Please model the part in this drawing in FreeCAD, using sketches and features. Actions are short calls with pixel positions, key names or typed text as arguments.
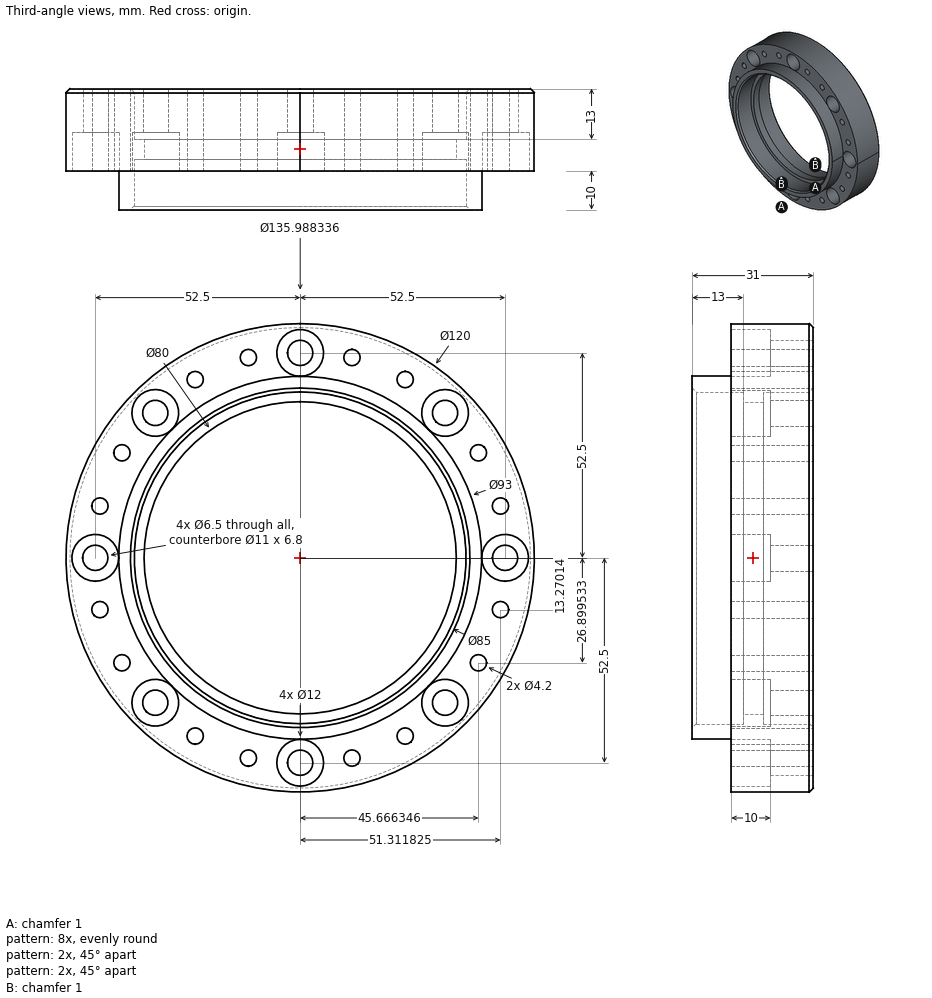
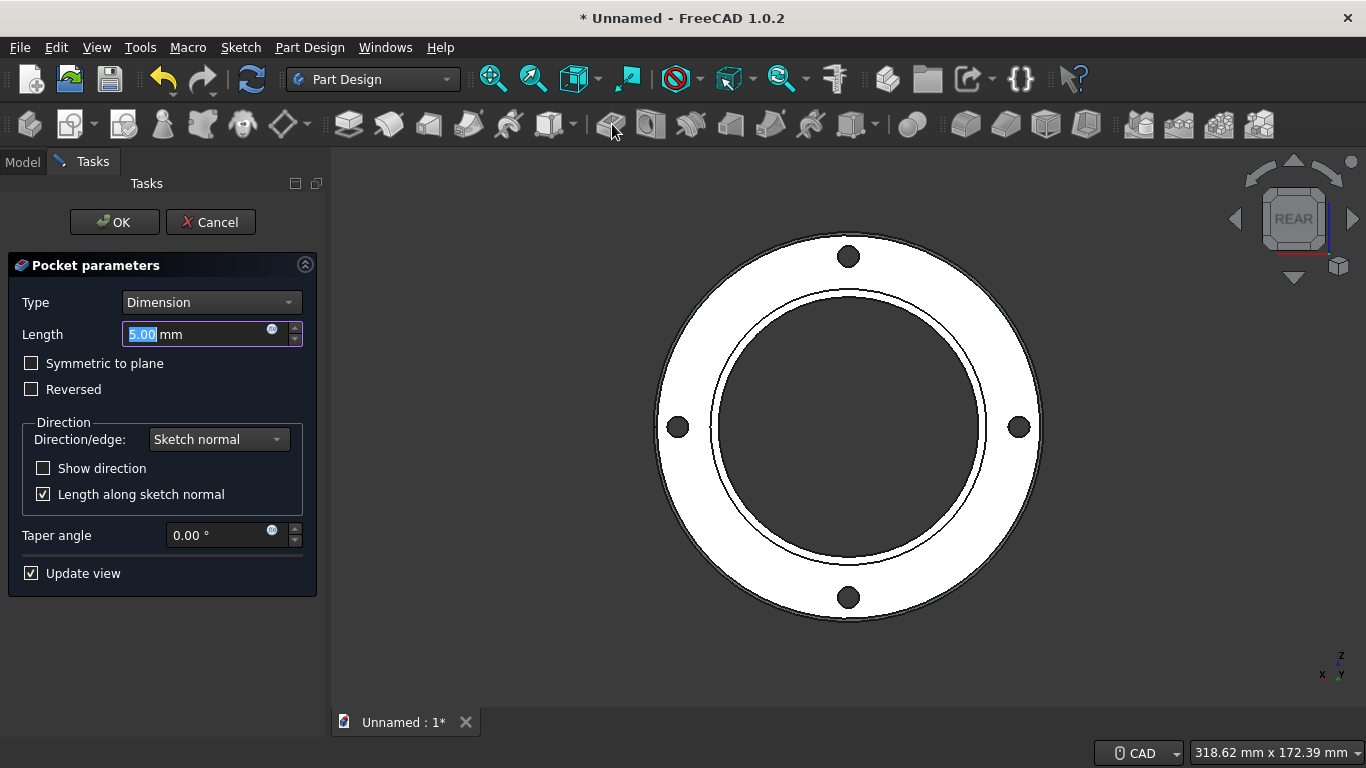
text(13)
key(Tab)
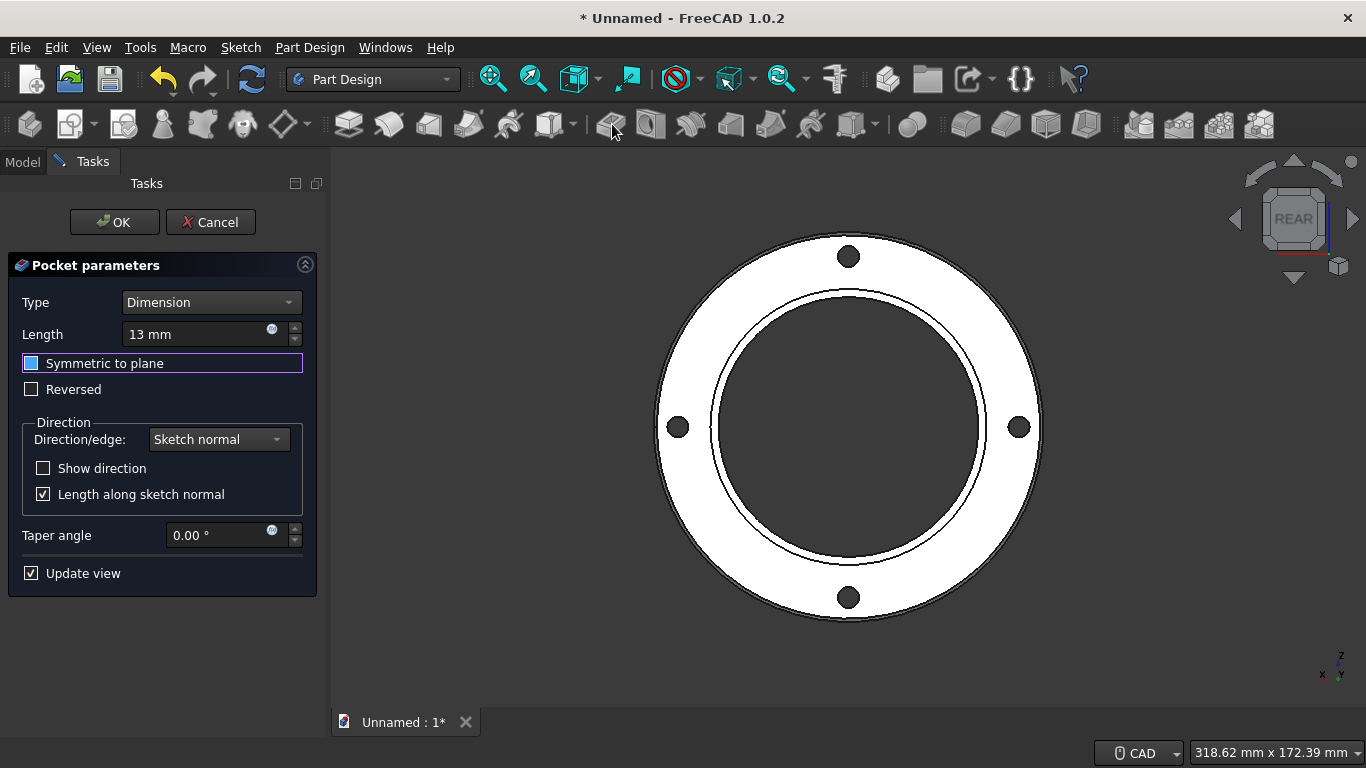
click(115, 222)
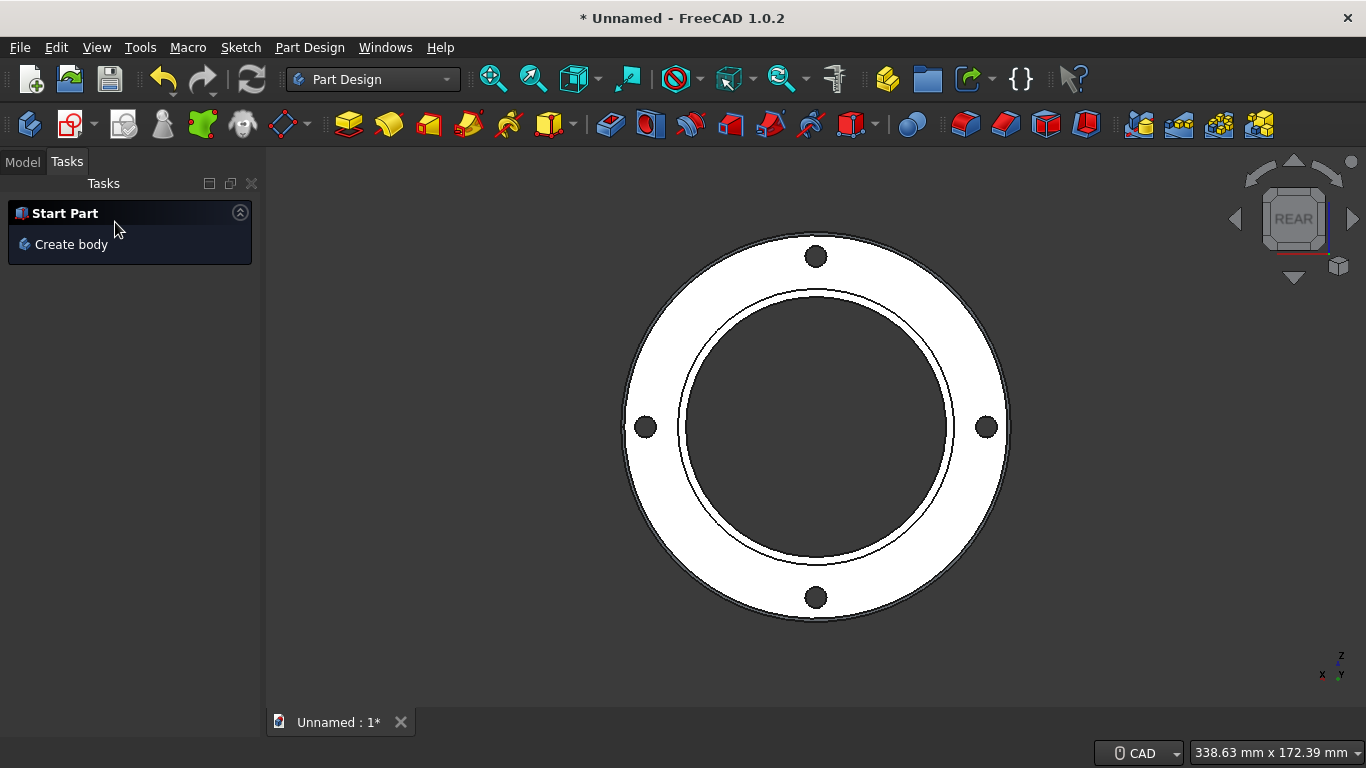
click(23, 161)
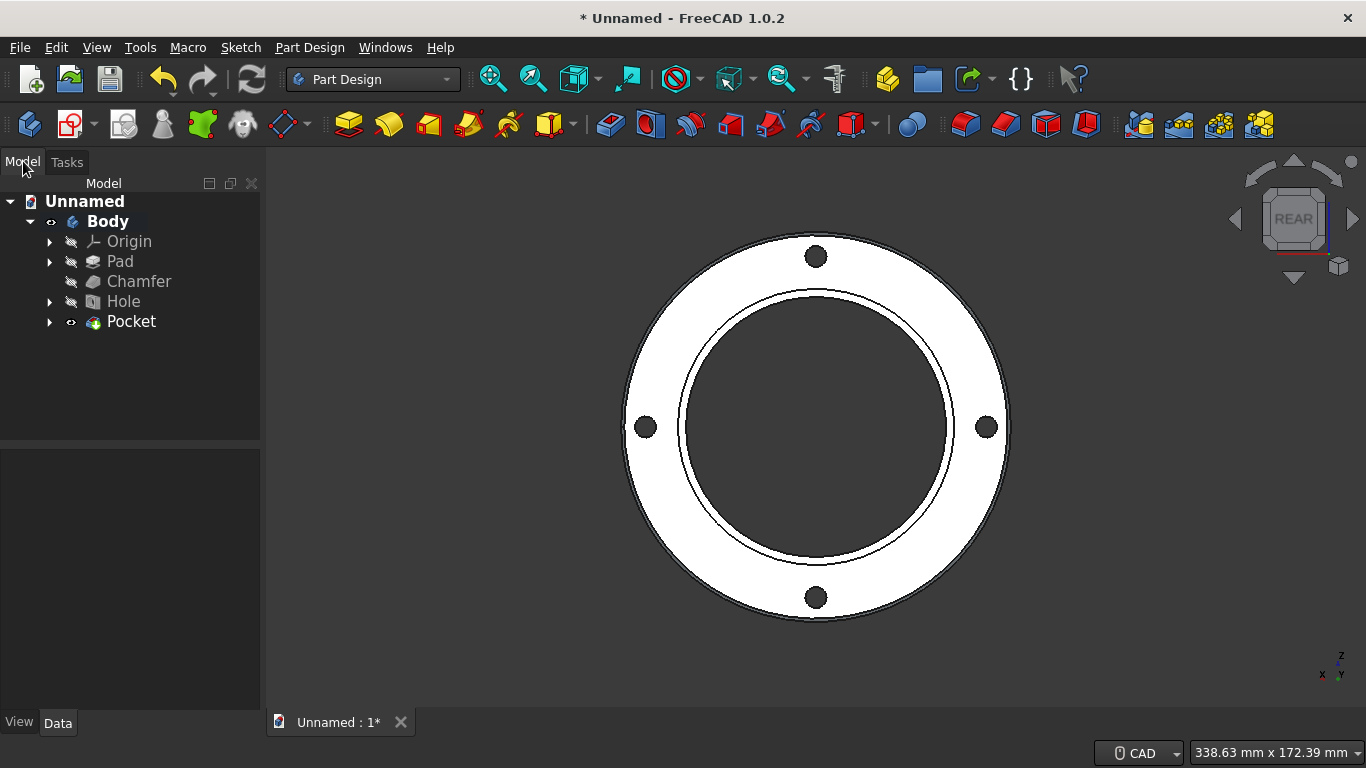
click(50, 242)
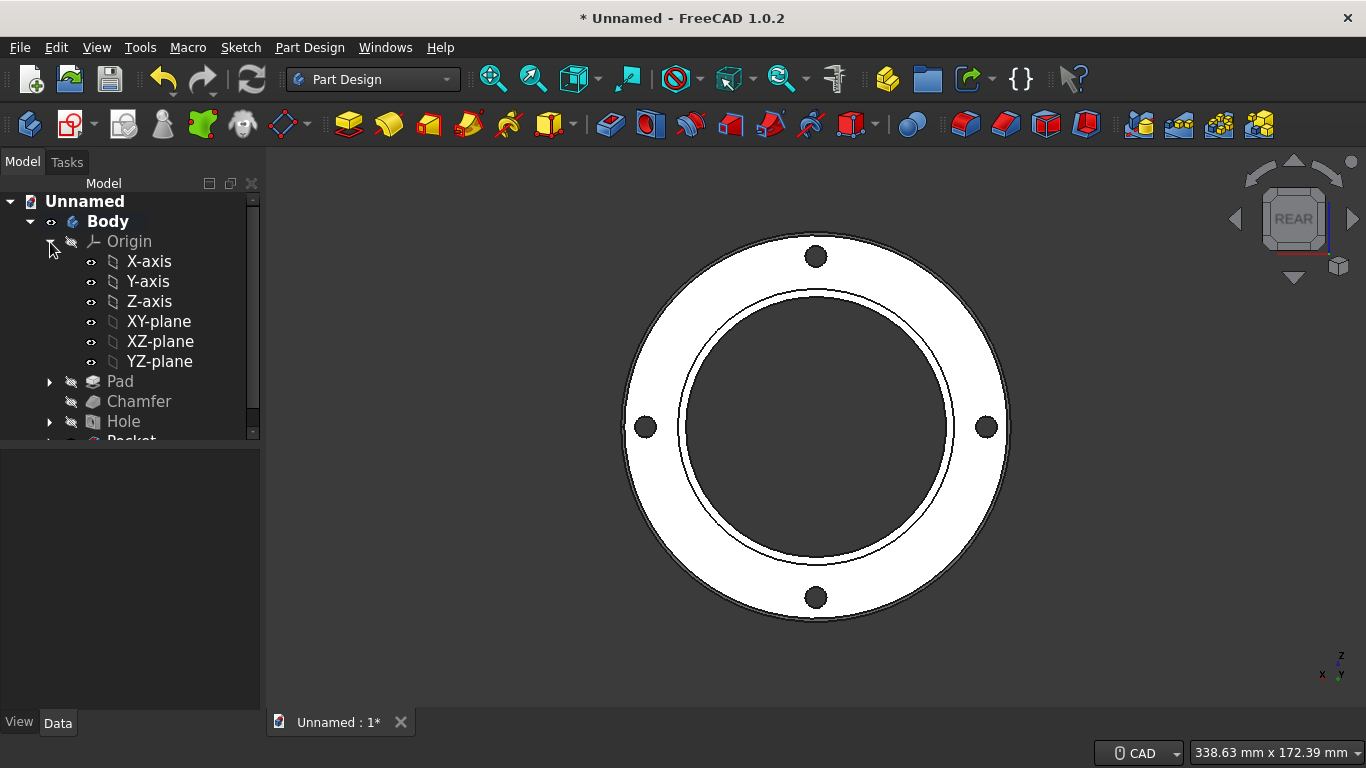
click(136, 342)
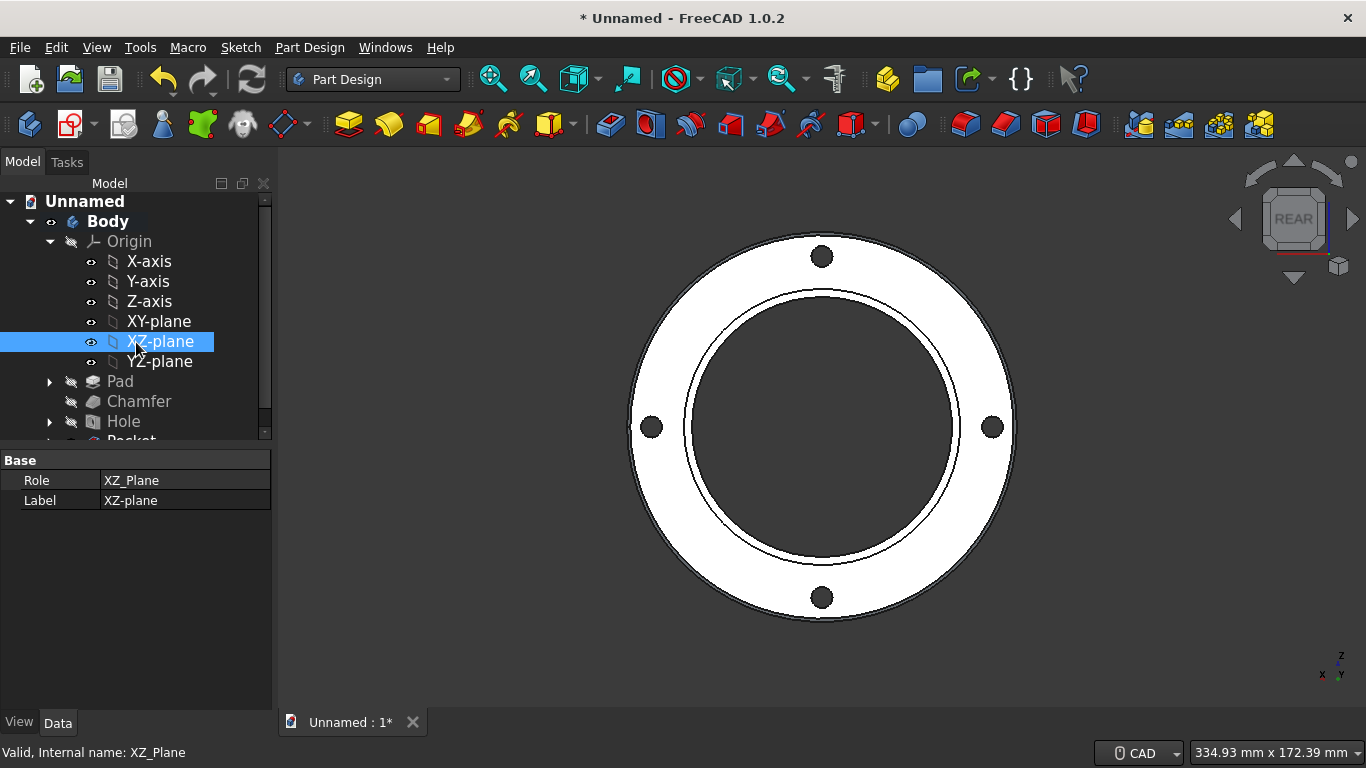
click(284, 124)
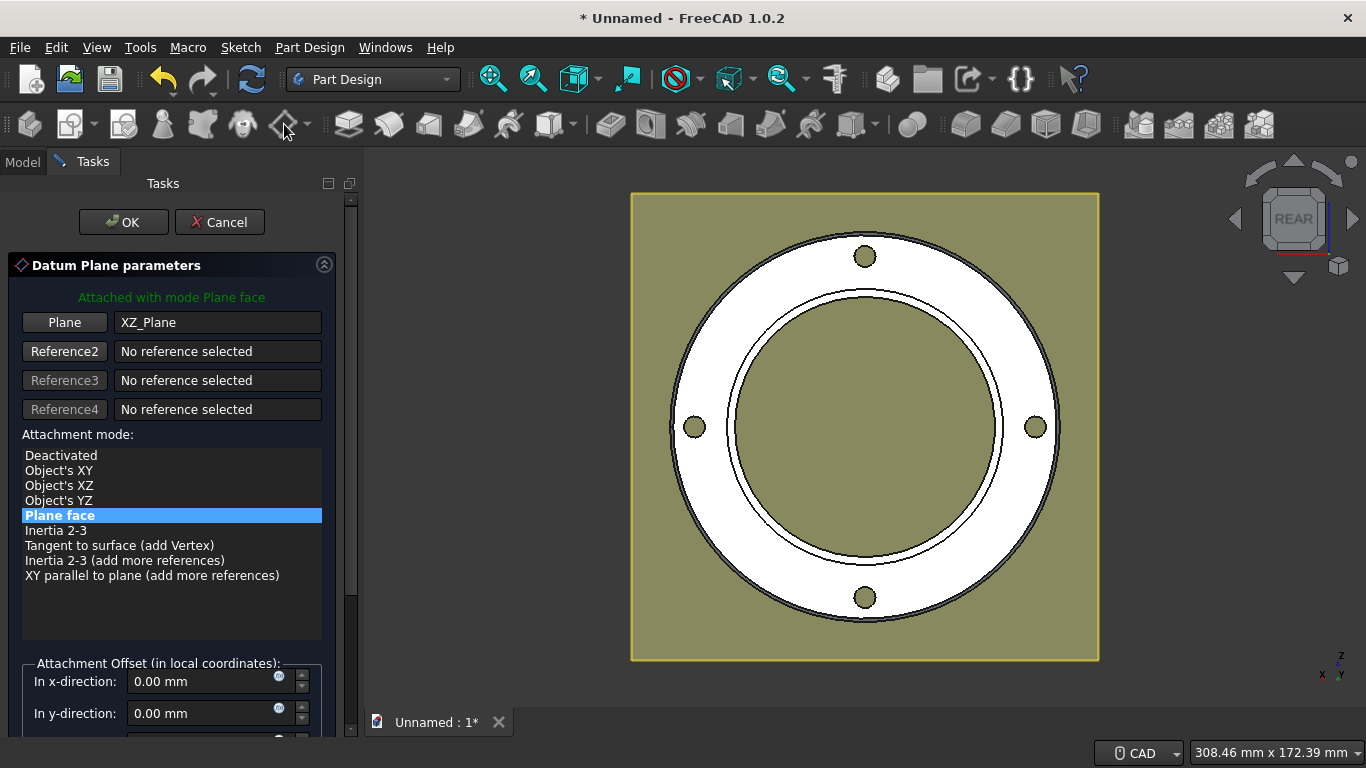
scroll(351, 464, down, 2)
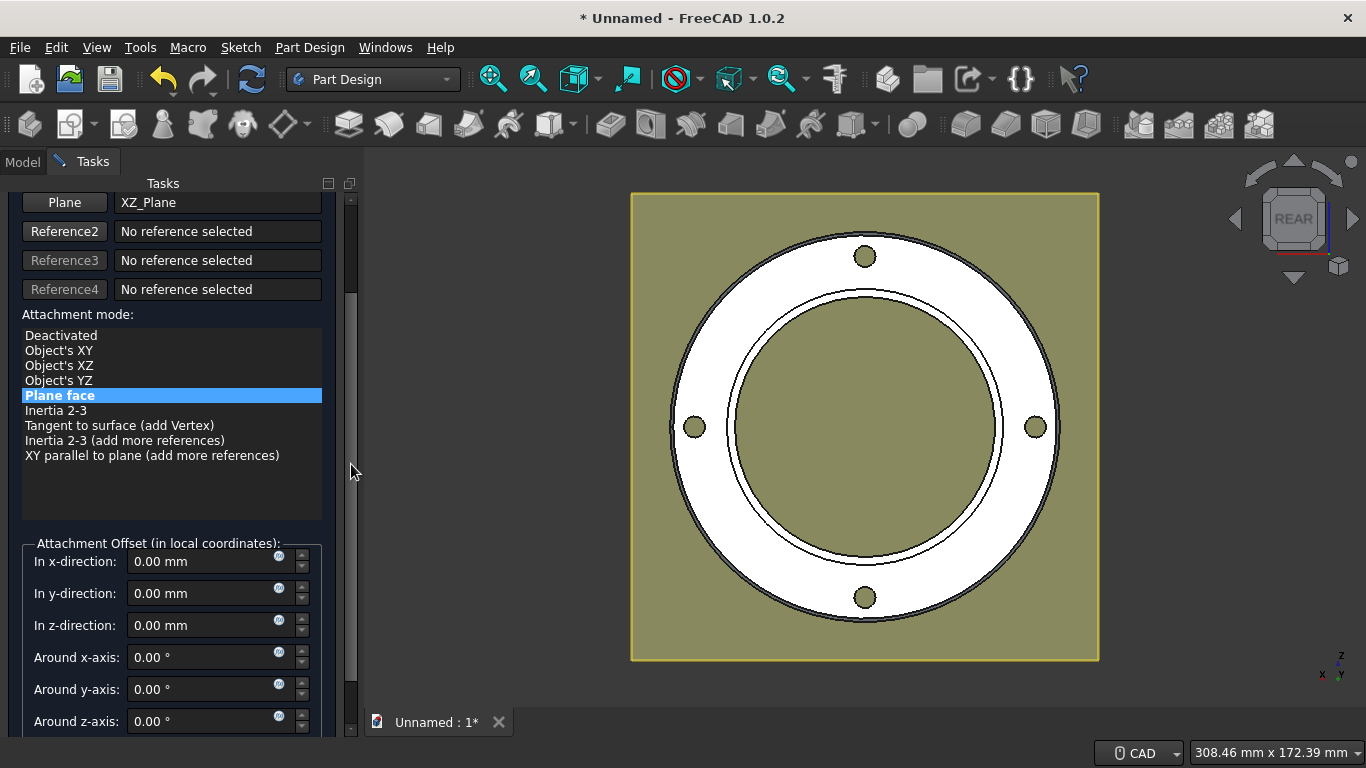
triple_click(210, 625)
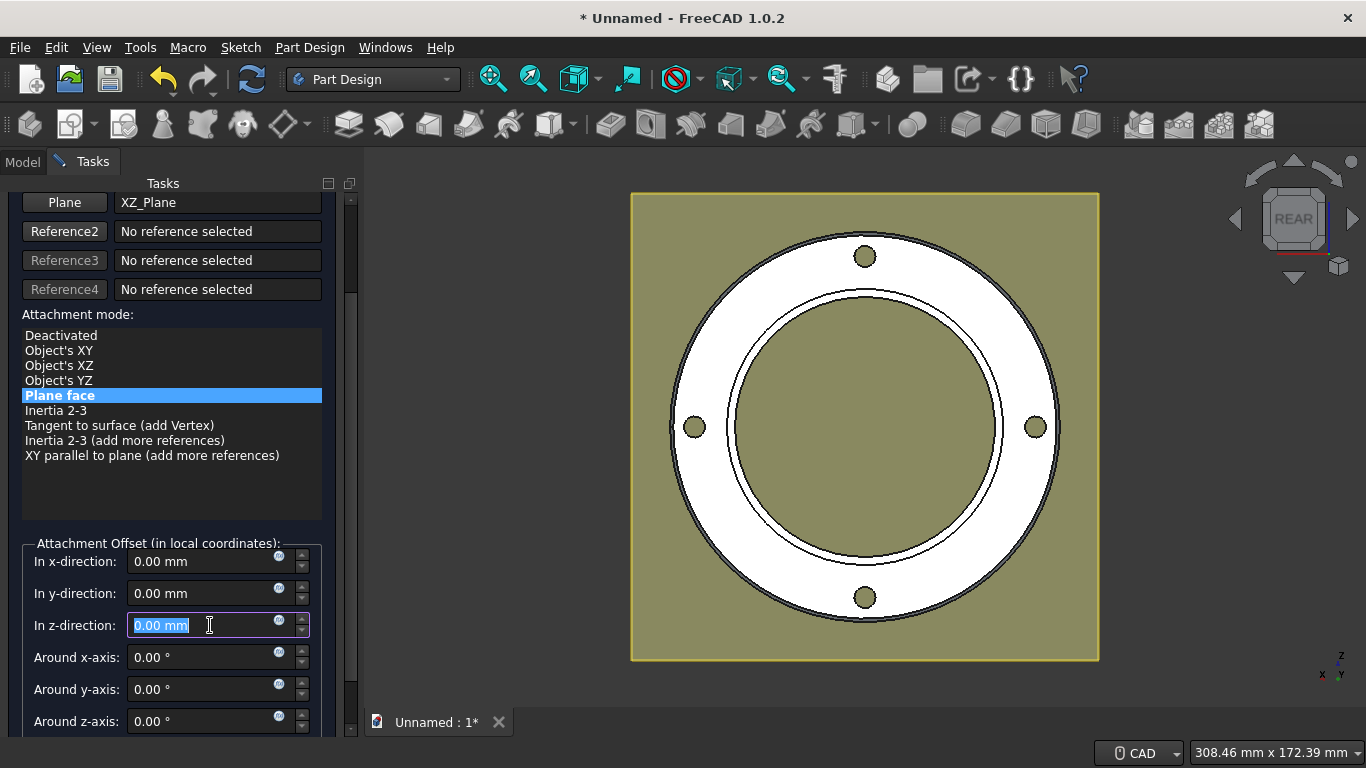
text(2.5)
key(Tab)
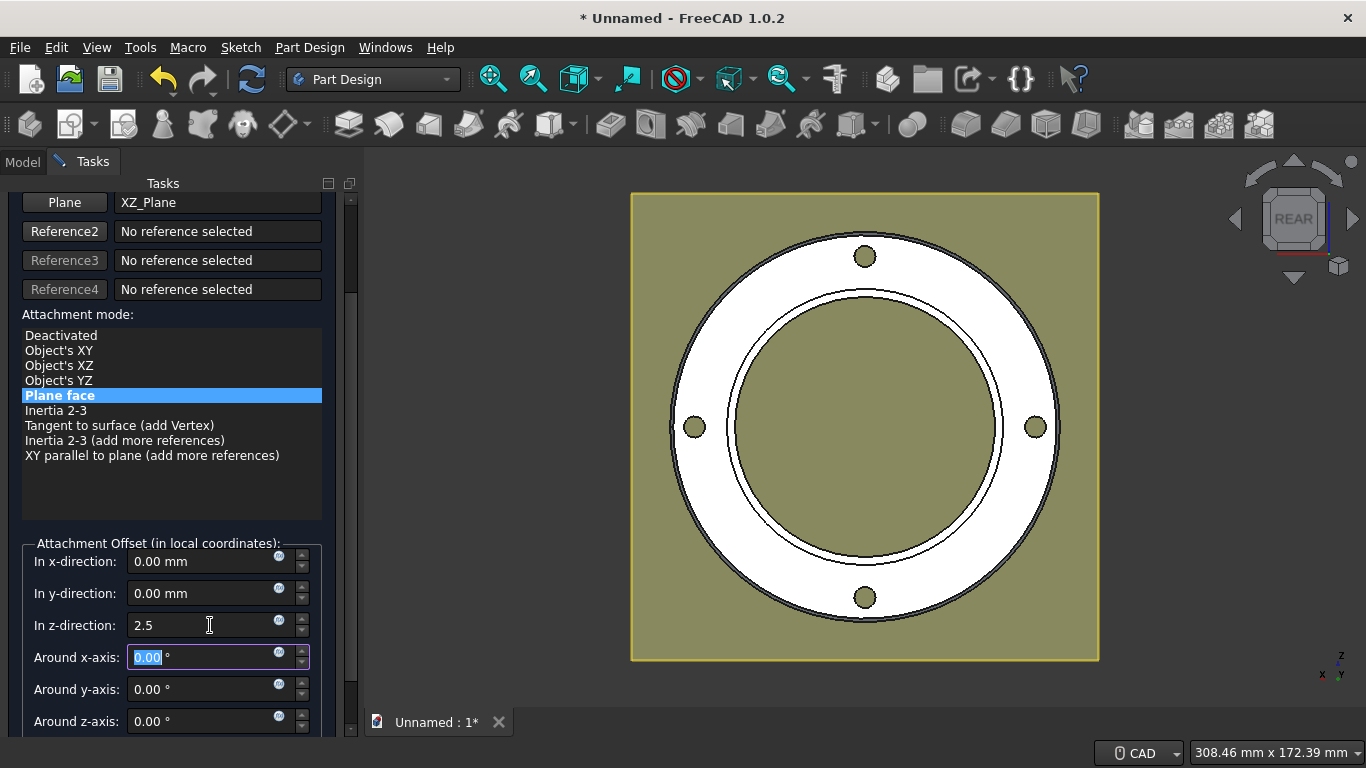
scroll(351, 464, up, 3)